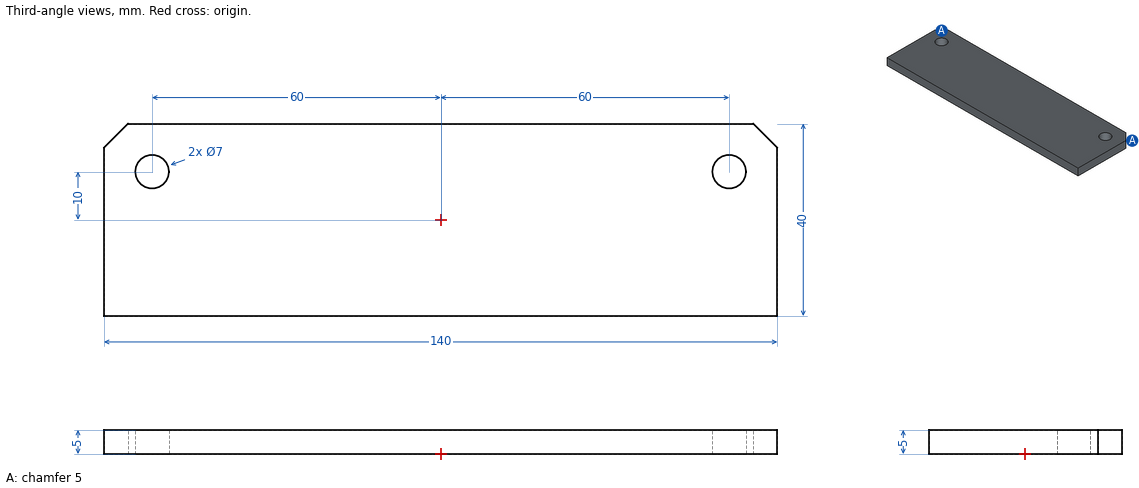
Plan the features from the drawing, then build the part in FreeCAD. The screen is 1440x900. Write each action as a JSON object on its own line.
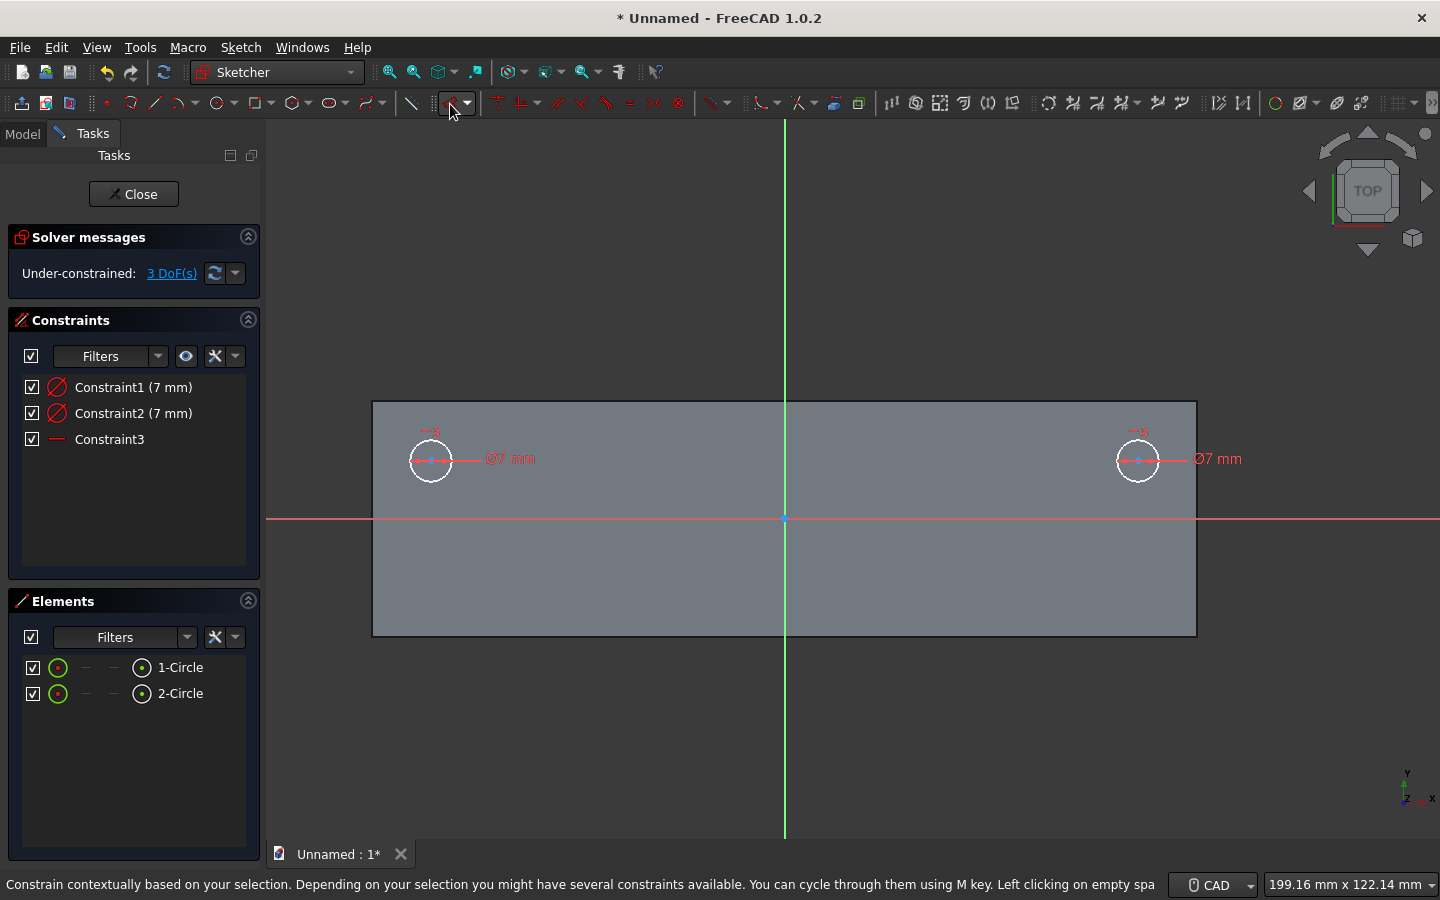
{"action": "left_click", "coordinate": [431, 461]}
{"action": "left_click", "coordinate": [608, 553]}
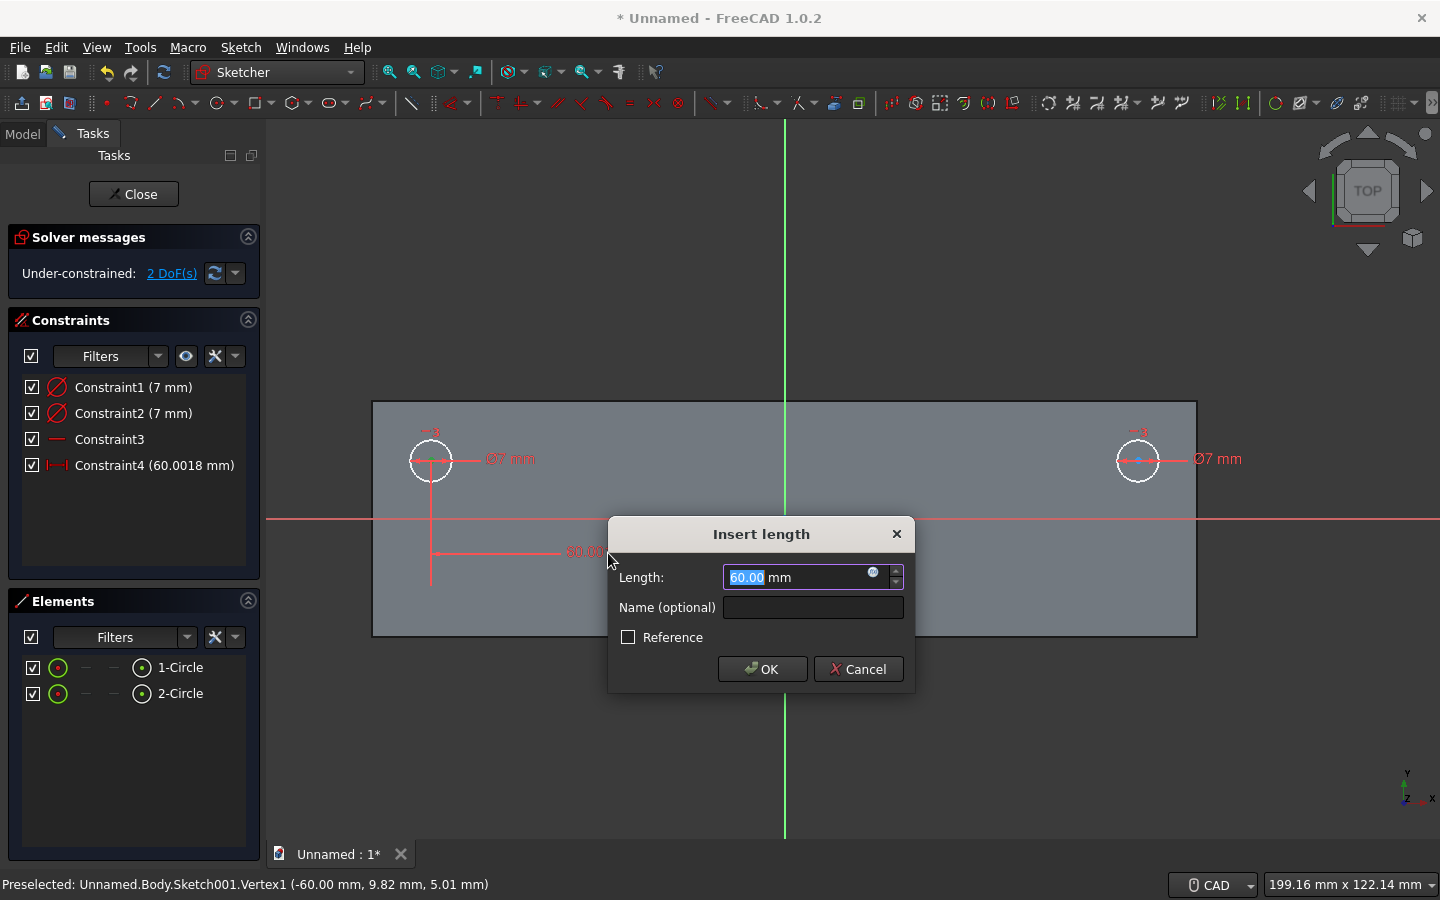
{"action": "type", "text": "60"}
{"action": "key", "text": "Return"}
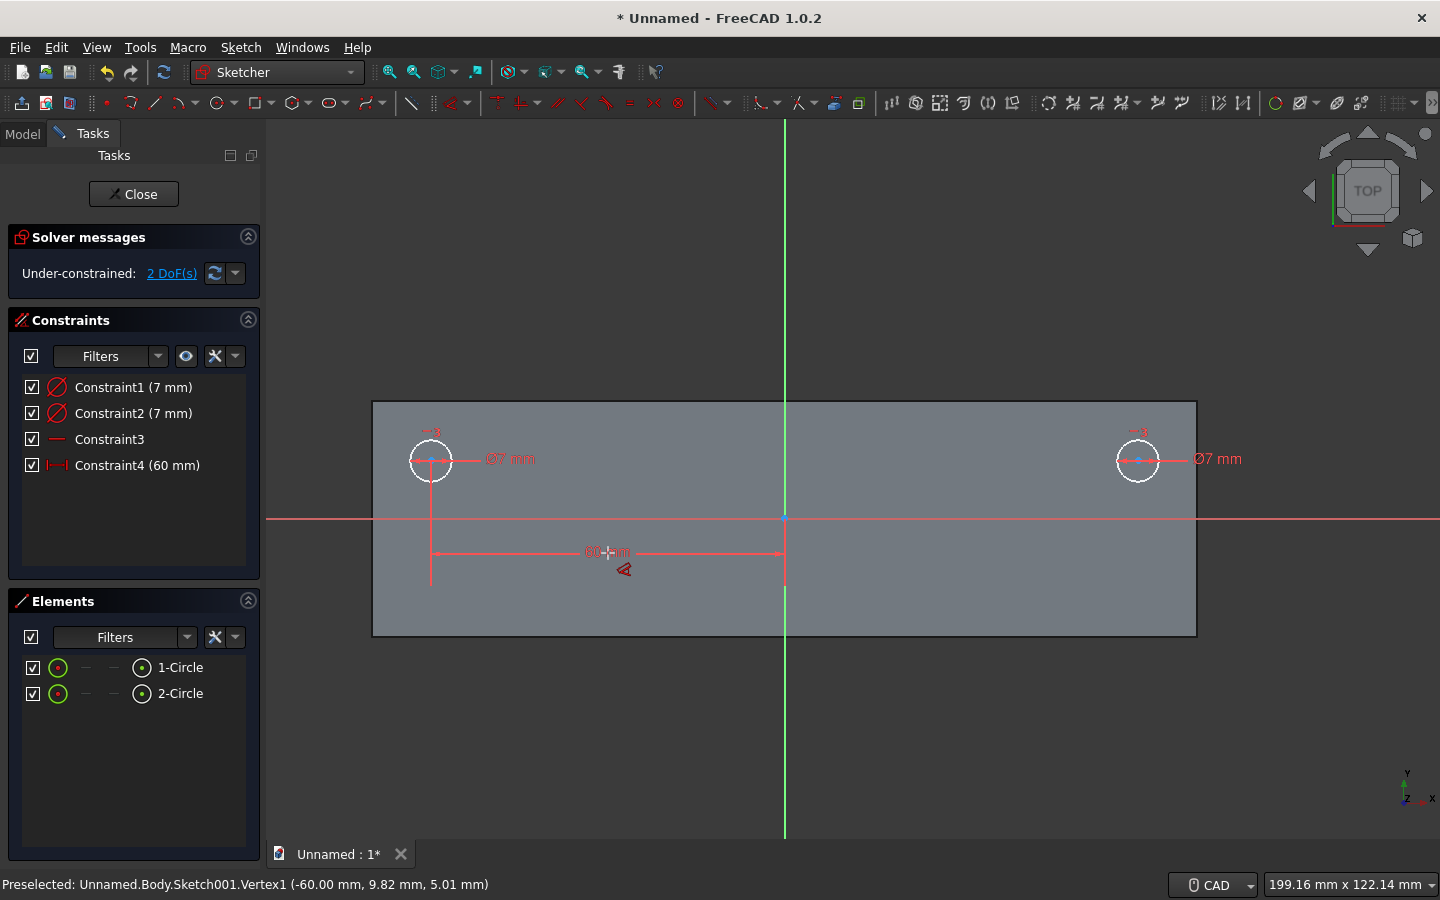
{"action": "left_click", "coordinate": [431, 461]}
{"action": "left_click", "coordinate": [397, 490]}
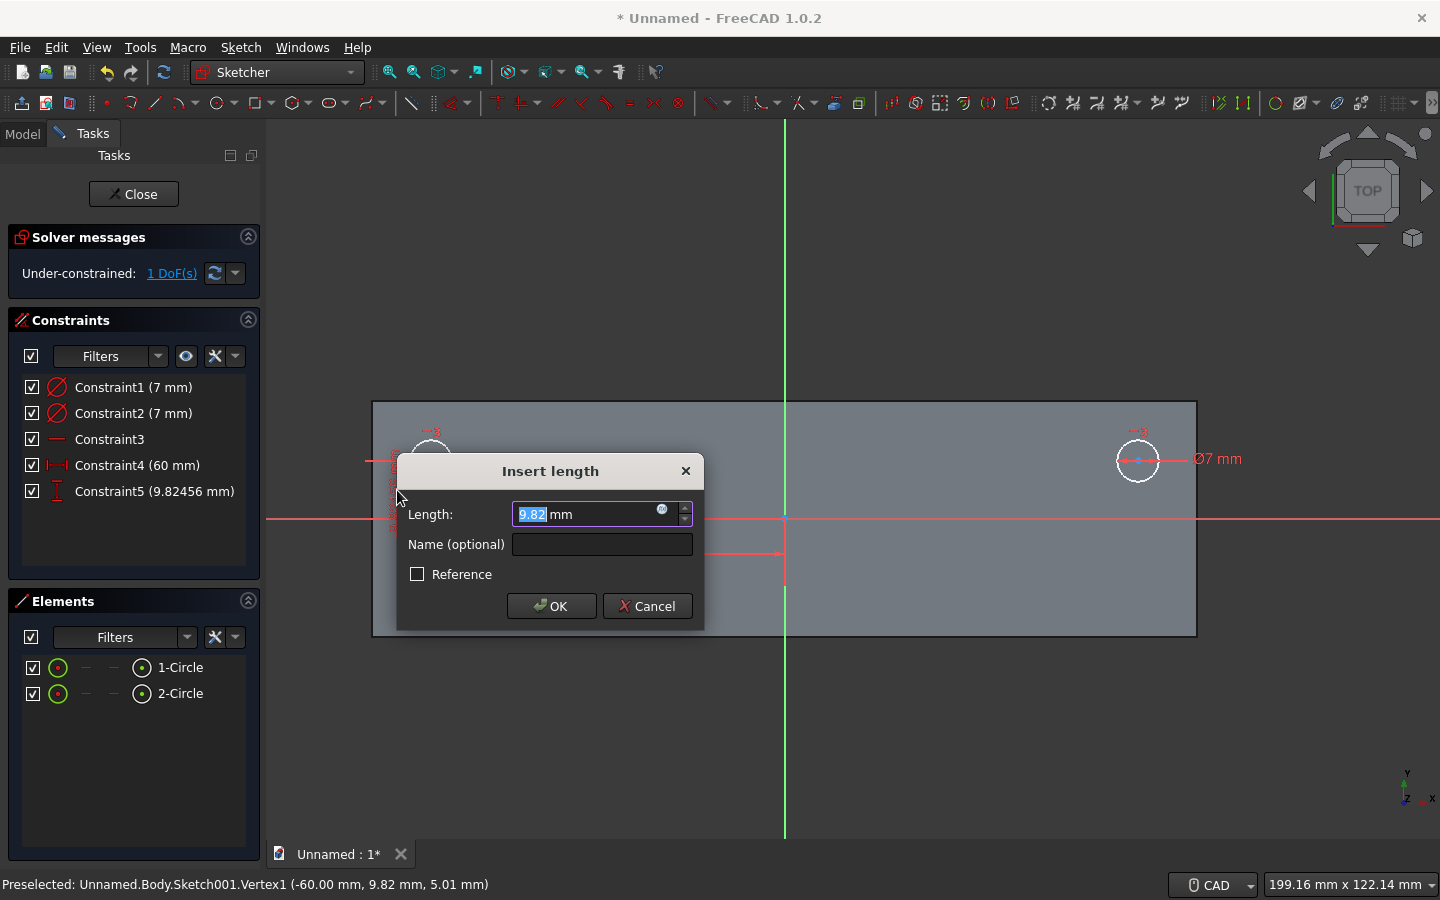
{"action": "type", "text": "10"}
{"action": "key", "text": "Return"}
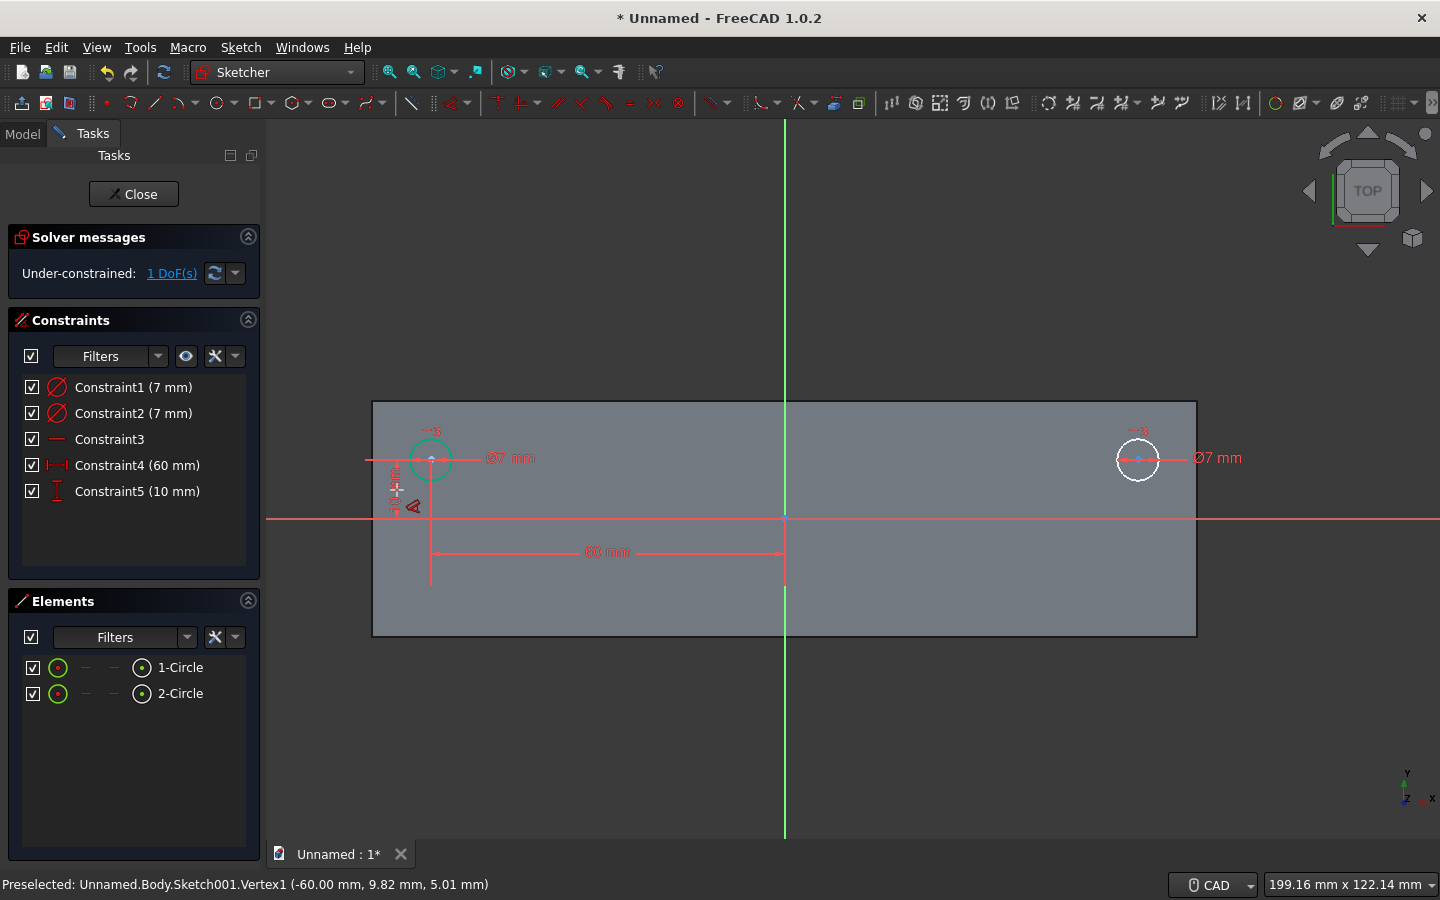
{"action": "left_click", "coordinate": [1138, 460]}
{"action": "left_click", "coordinate": [961, 553]}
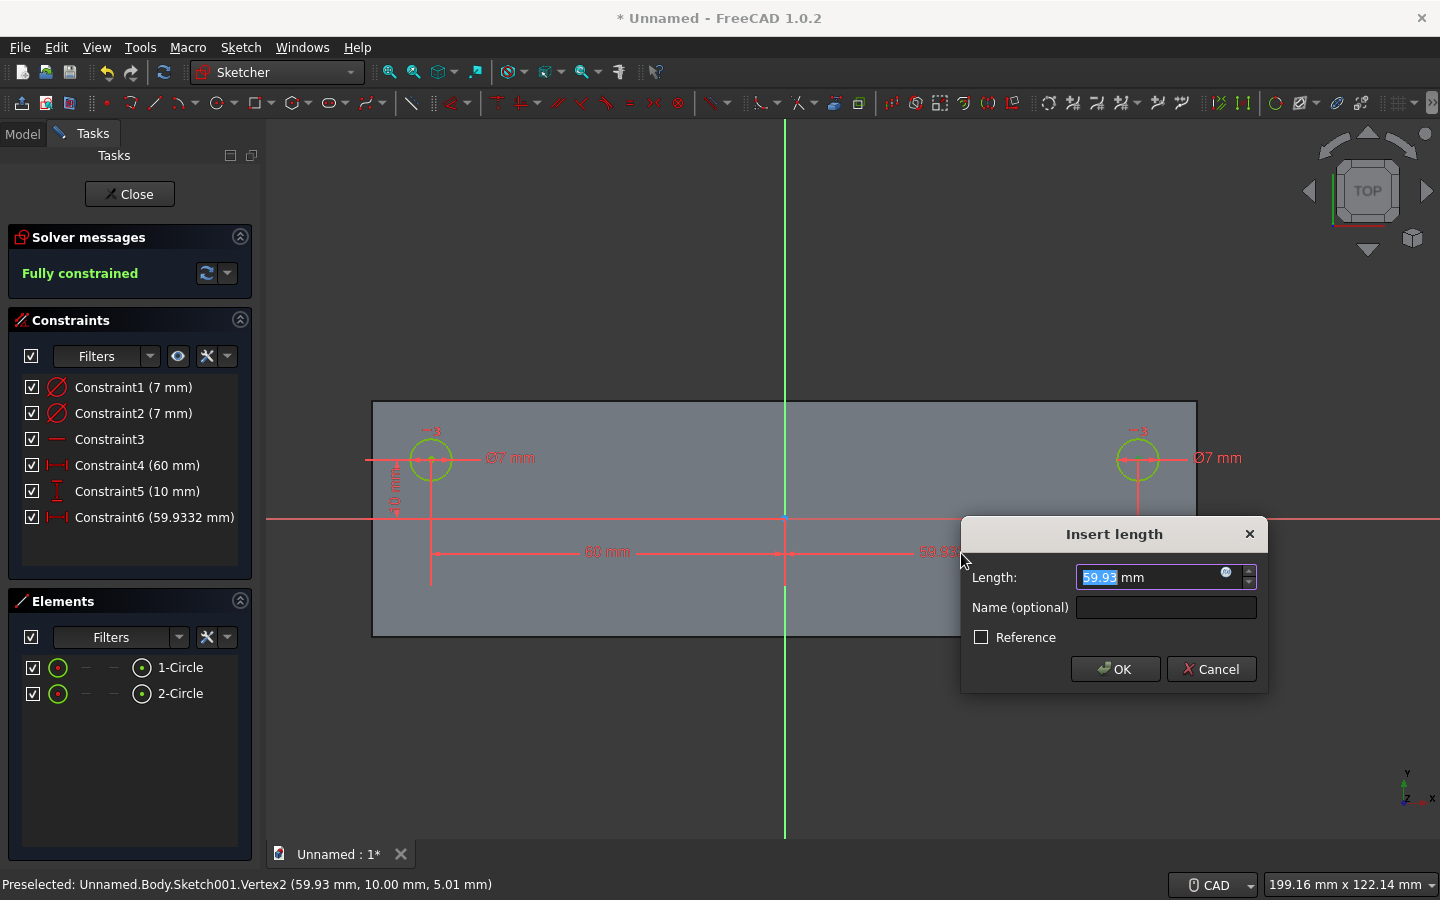
{"action": "type", "text": "60"}
{"action": "key", "text": "Return"}
{"action": "key", "text": "Escape"}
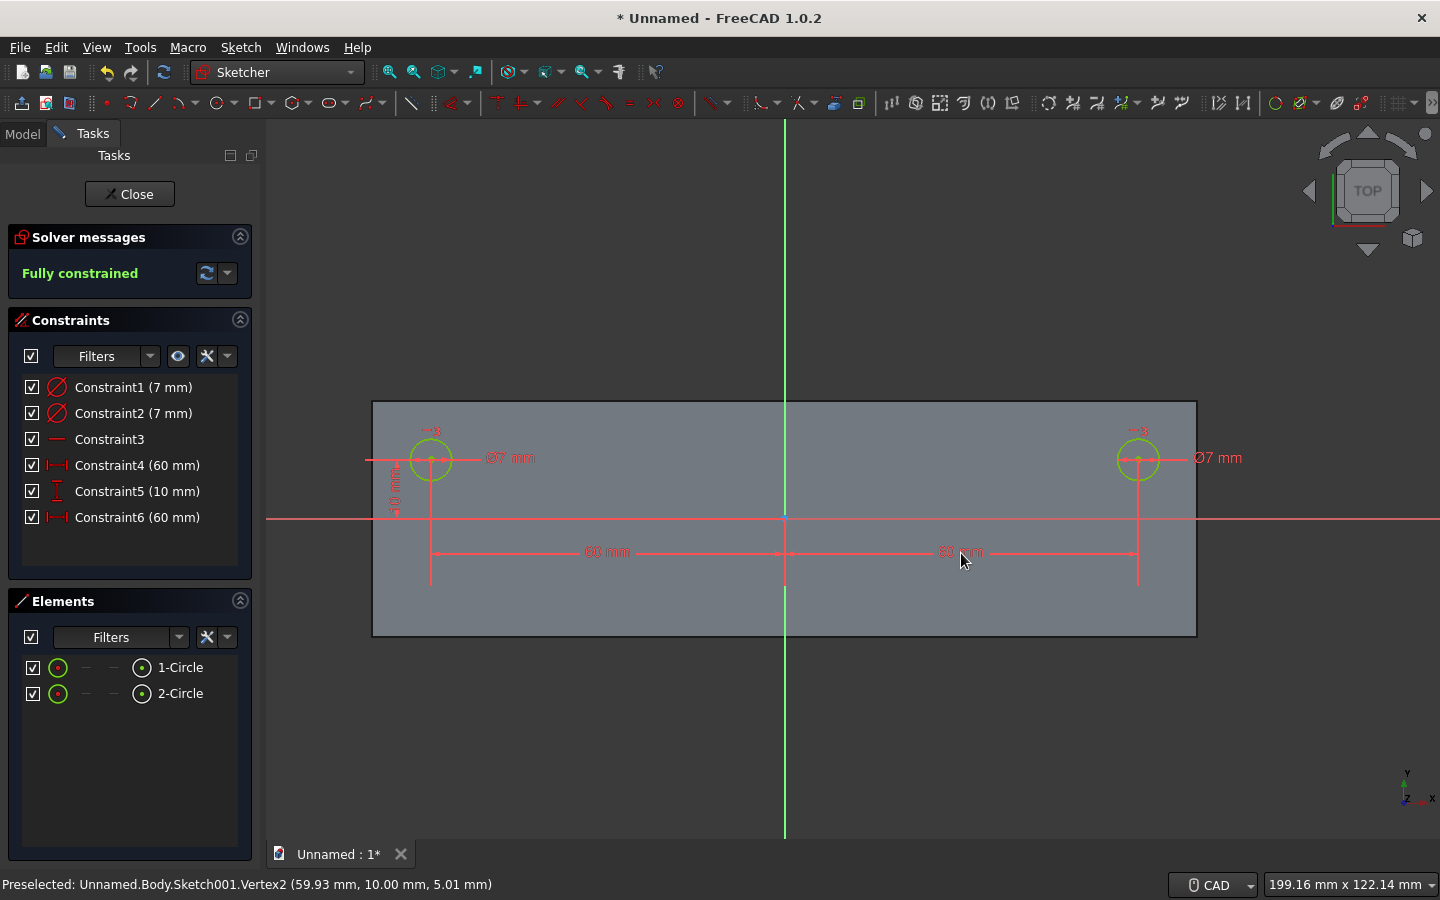
{"action": "left_click", "coordinate": [130, 194]}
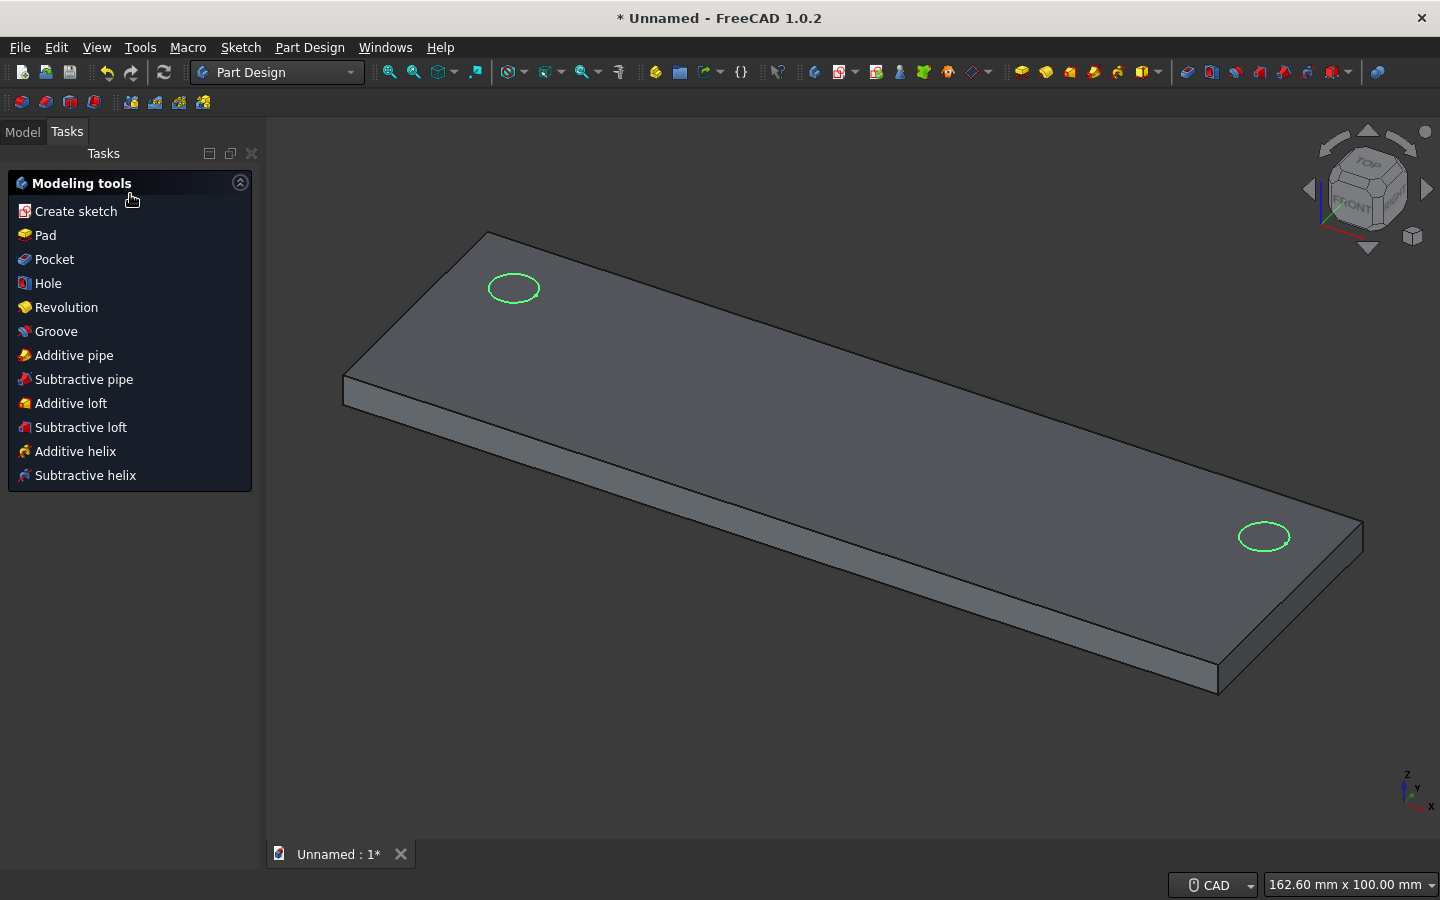
{"action": "left_click", "coordinate": [1188, 72]}